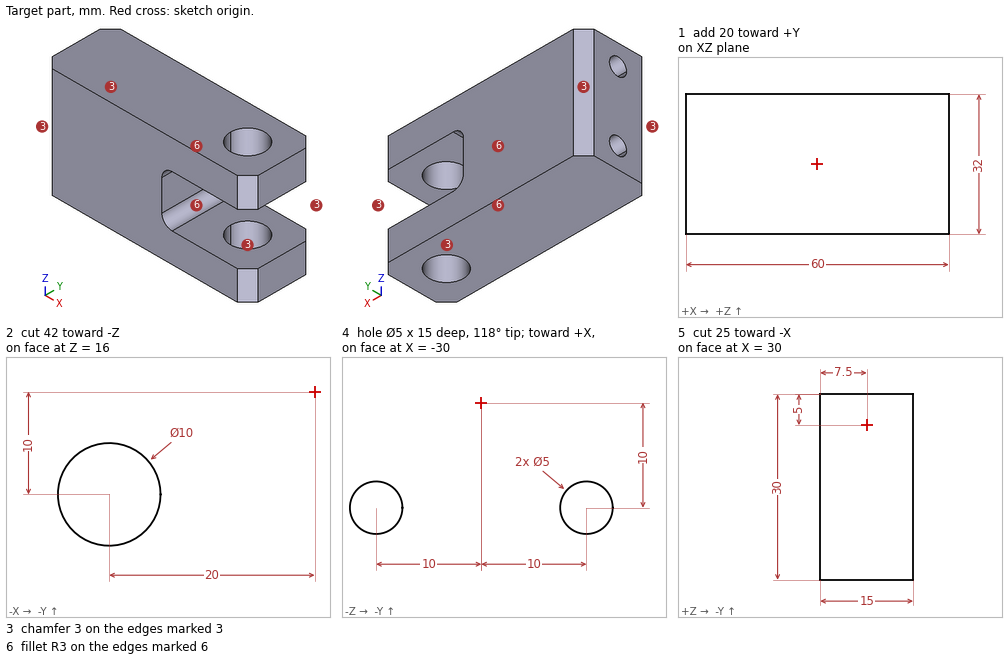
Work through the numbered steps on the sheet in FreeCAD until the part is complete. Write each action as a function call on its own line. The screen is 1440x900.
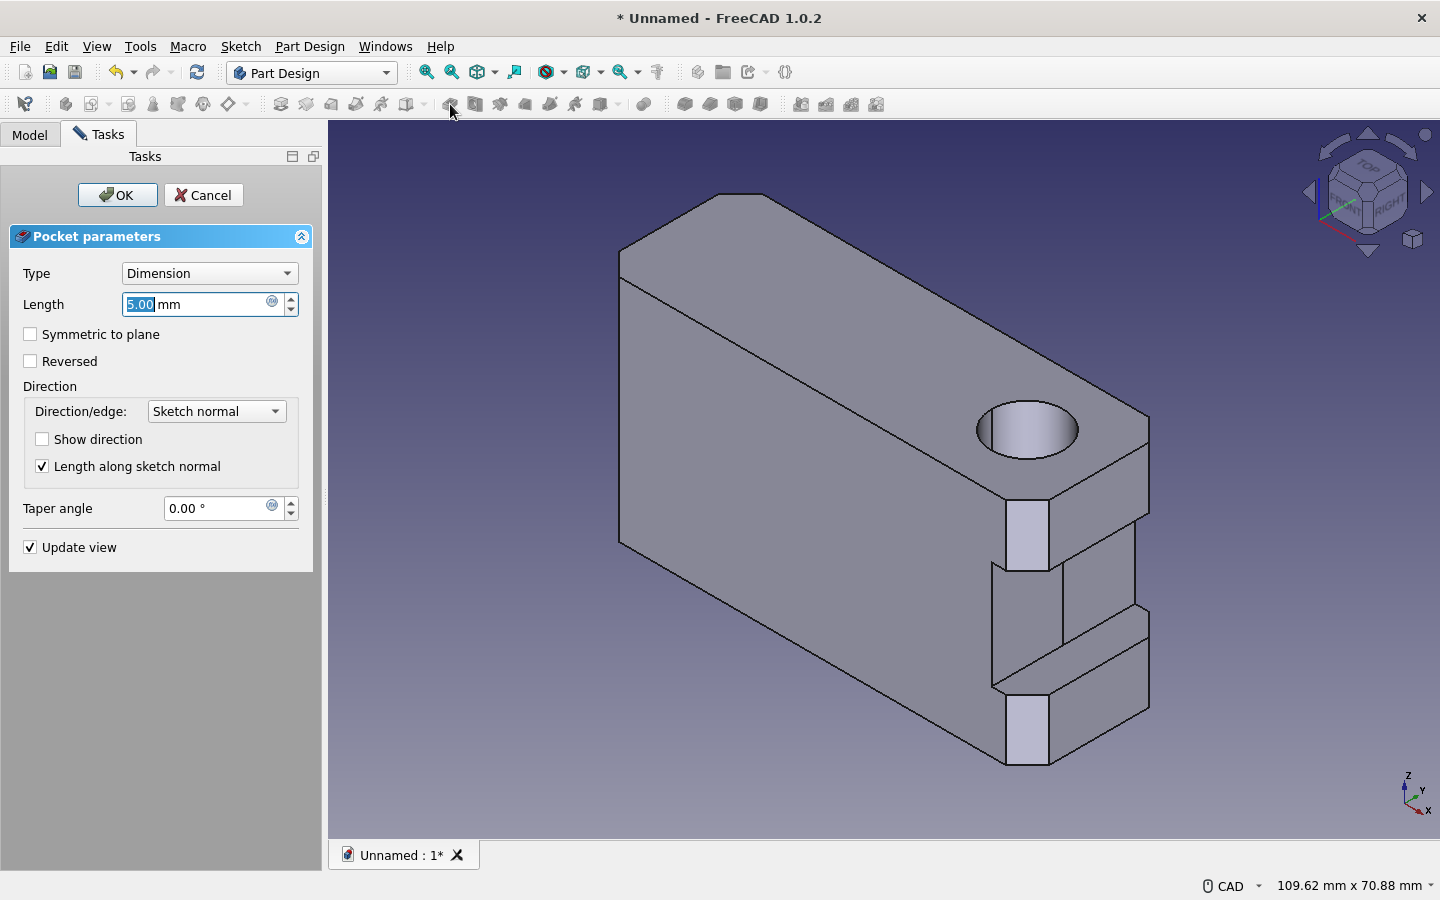
text(25)
key(Tab)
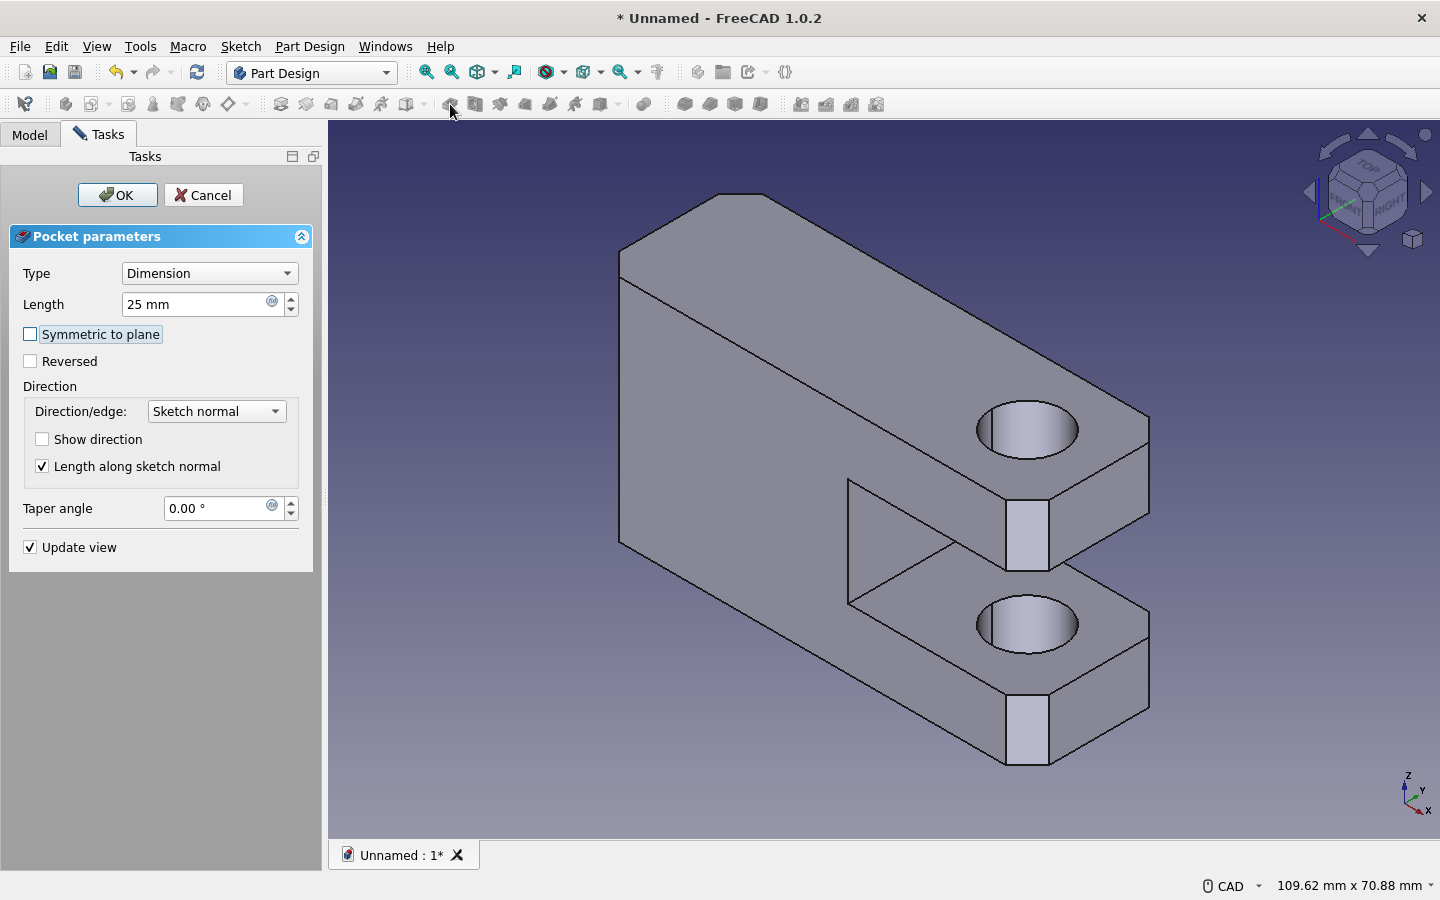
click(118, 195)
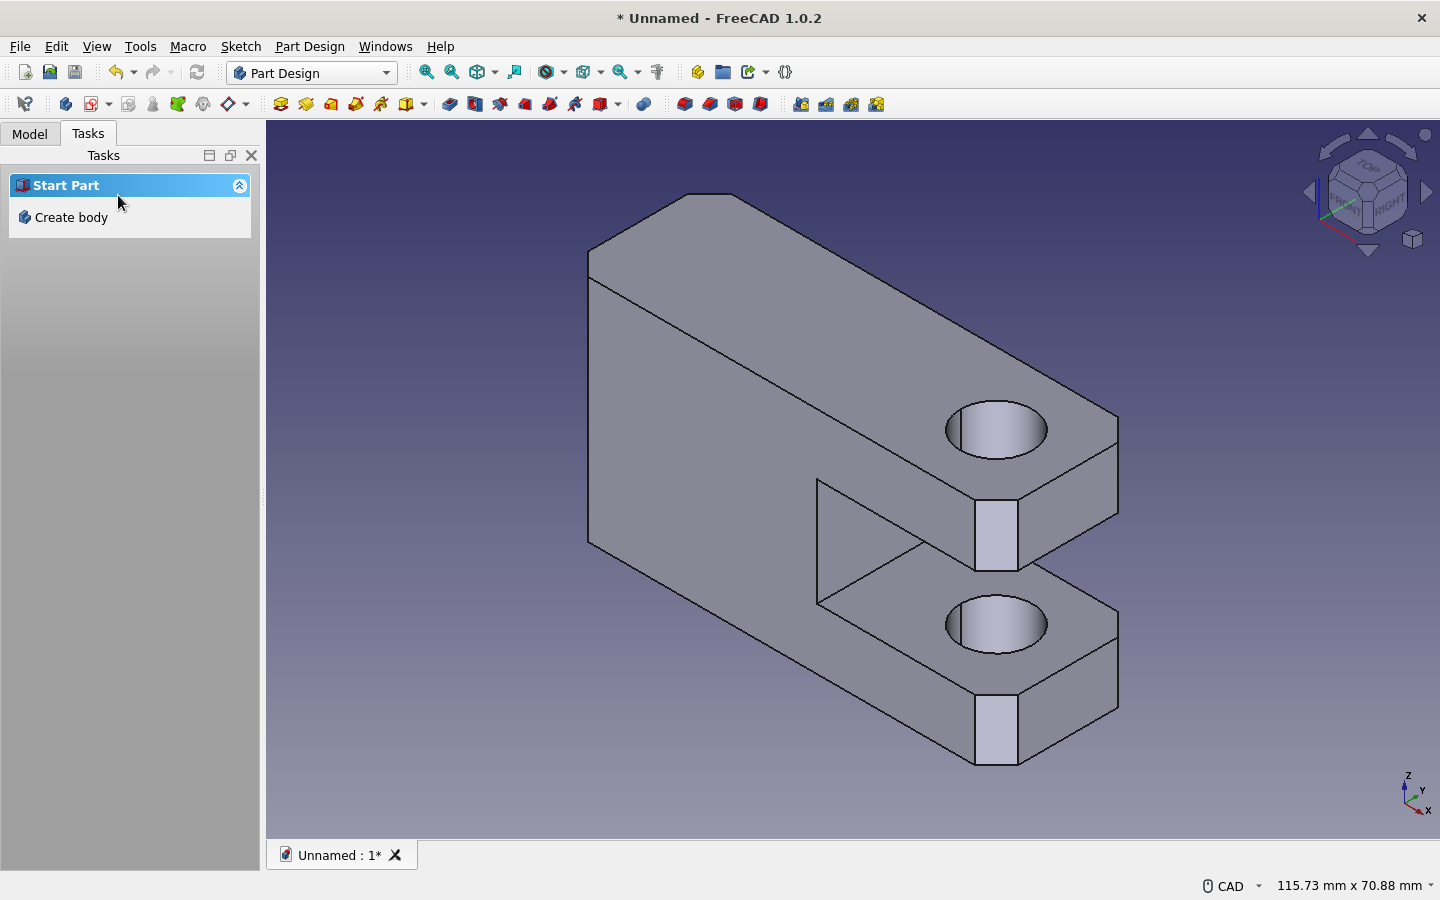
key(2)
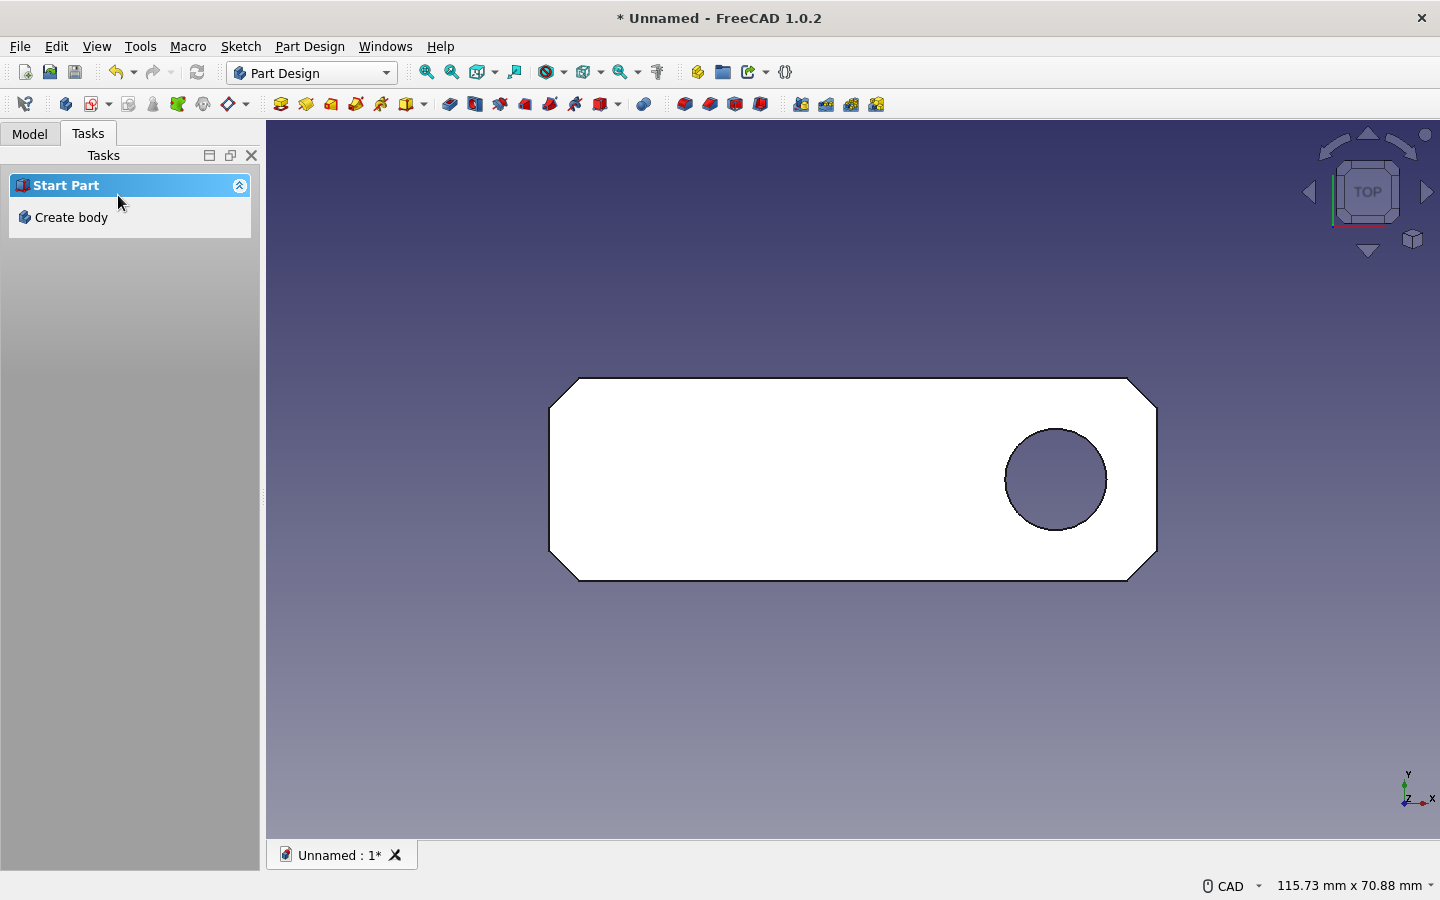
key(0)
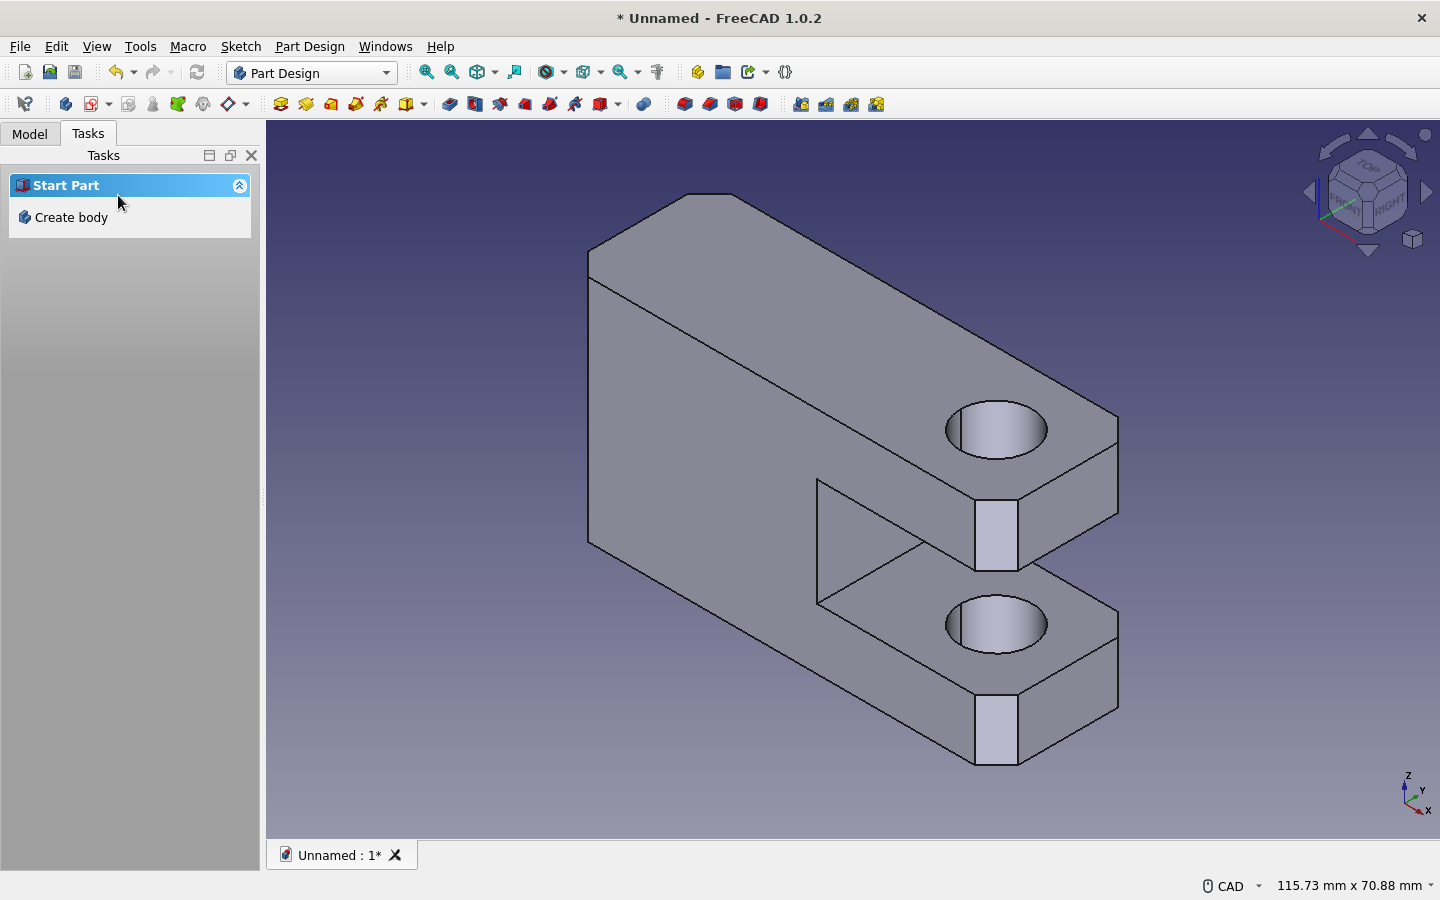
key(1)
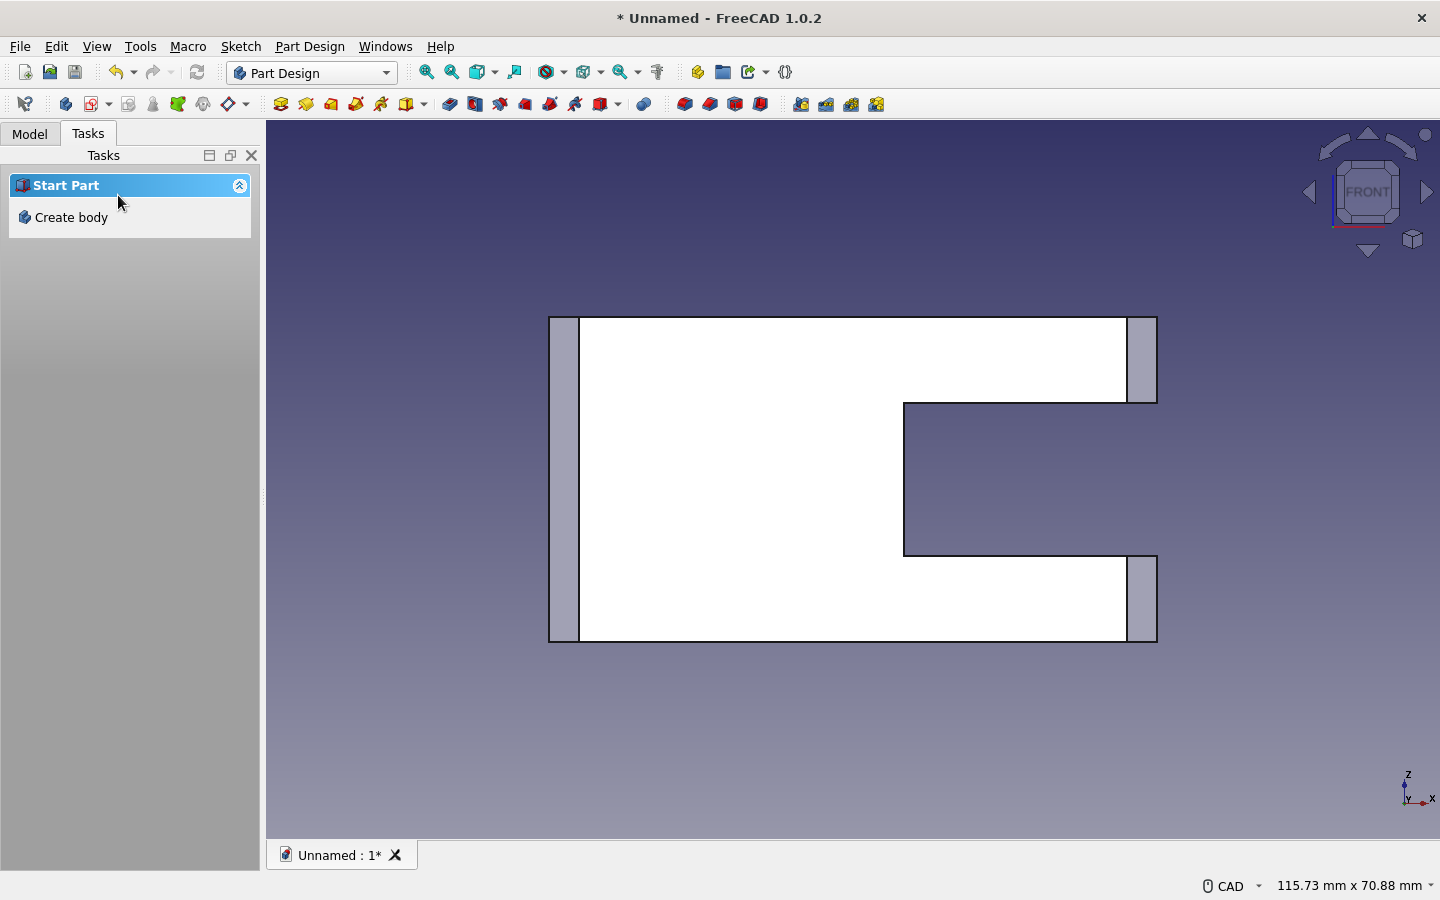
key(3)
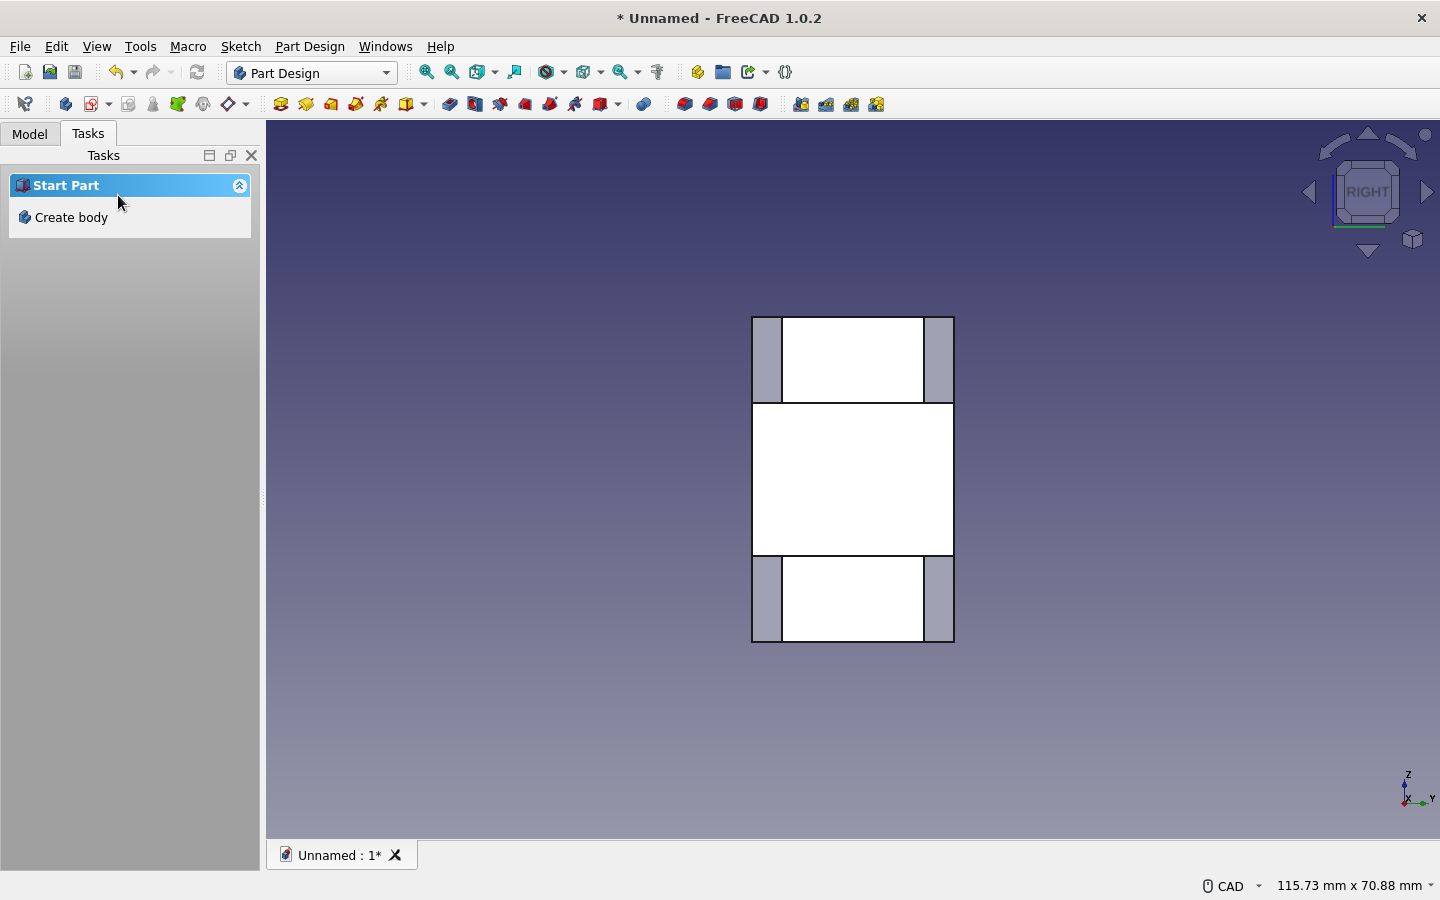
key(5)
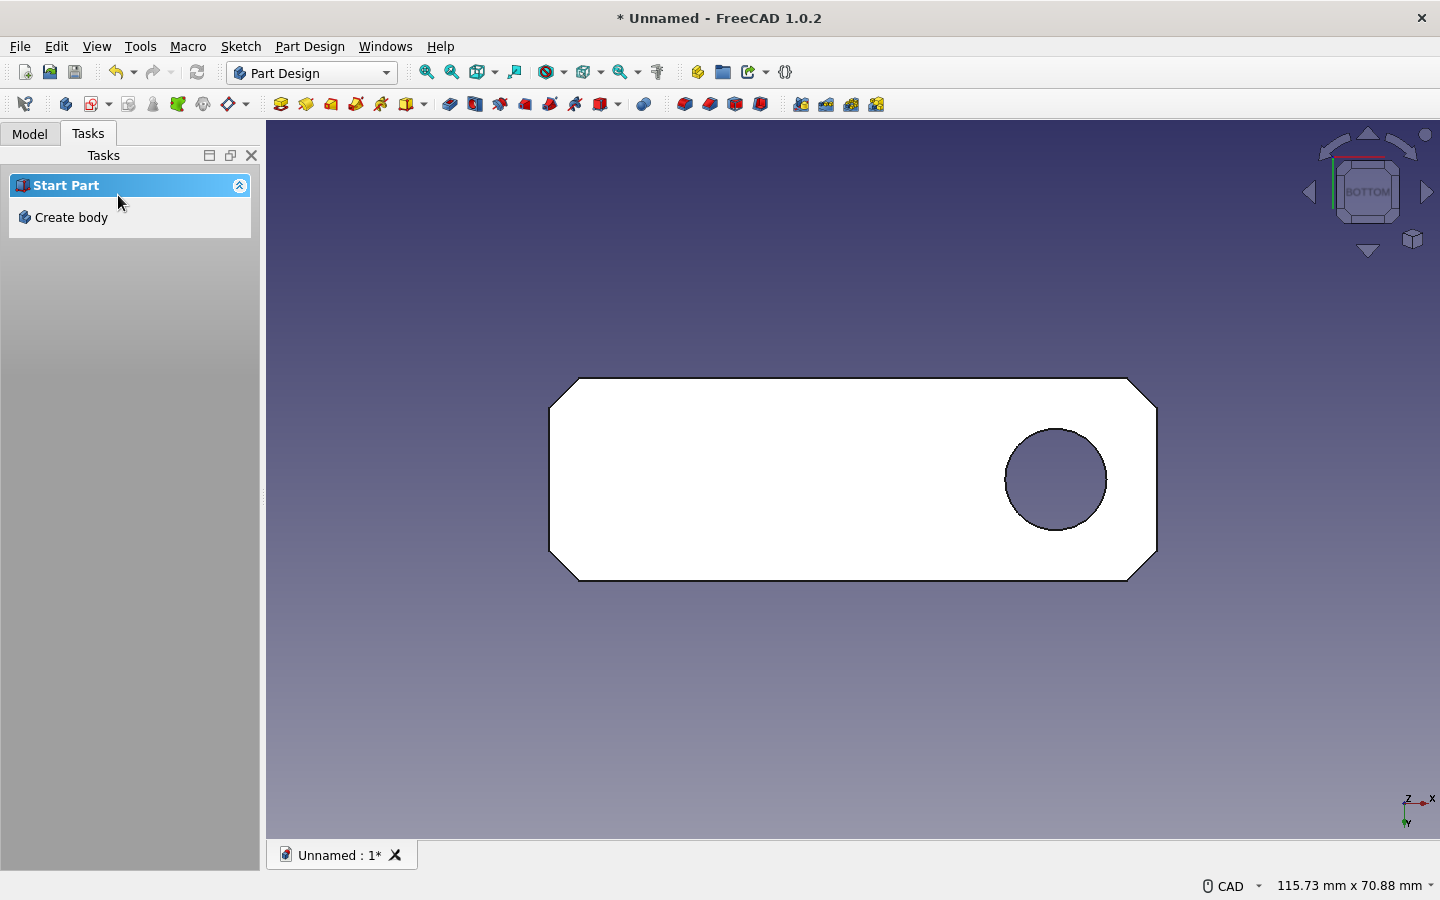
key(4)